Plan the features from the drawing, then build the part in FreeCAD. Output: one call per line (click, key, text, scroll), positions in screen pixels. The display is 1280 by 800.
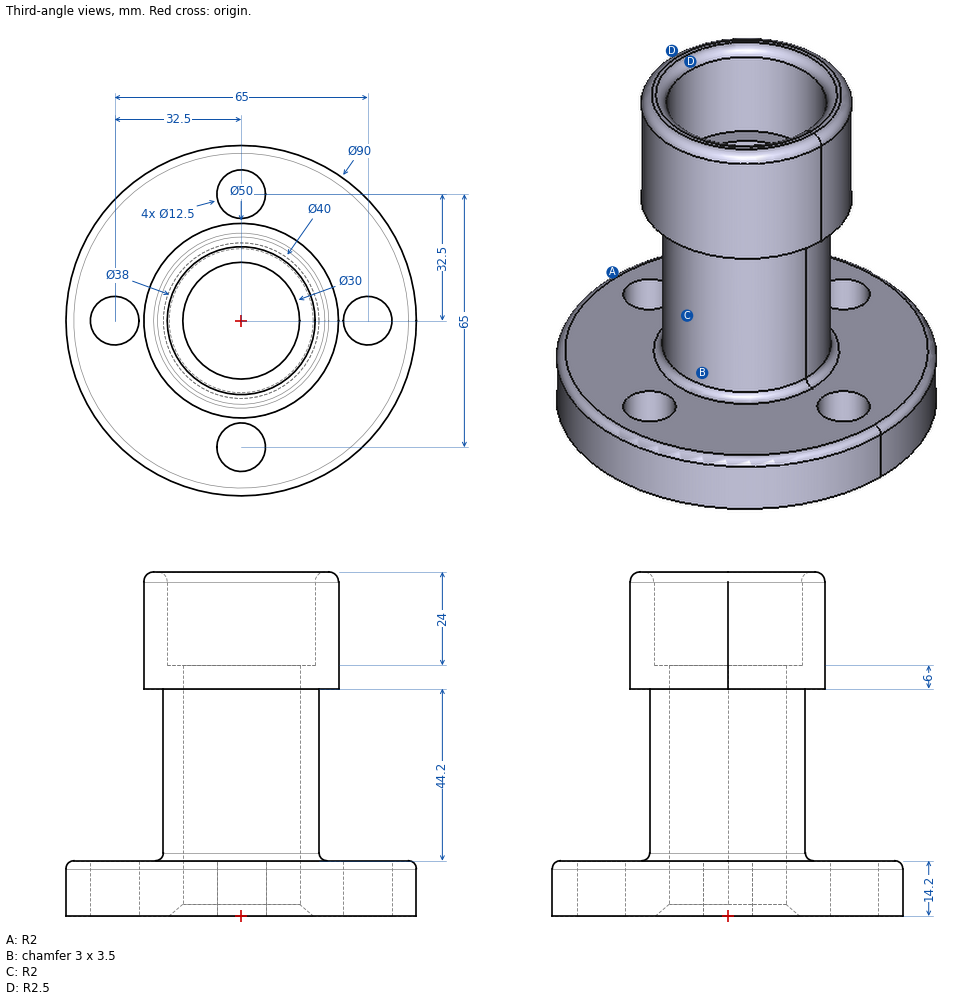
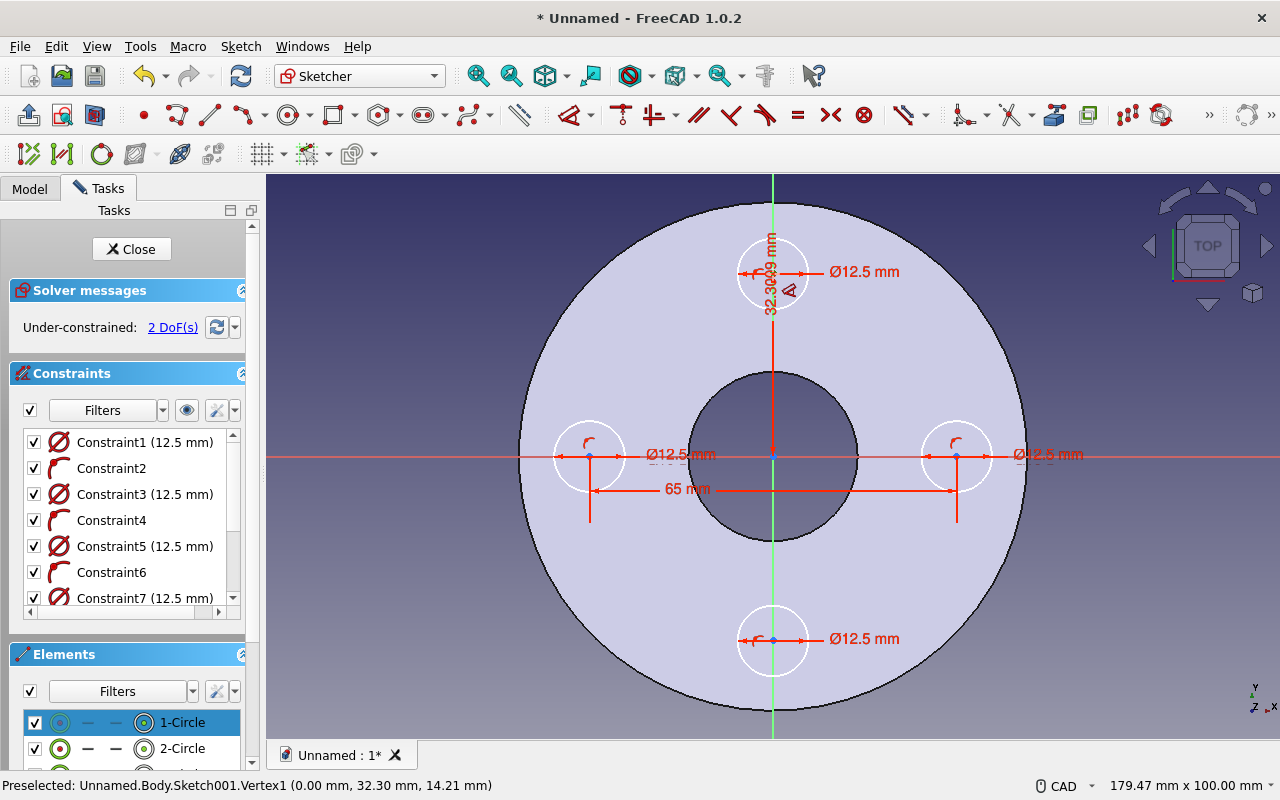
click(773, 641)
click(807, 373)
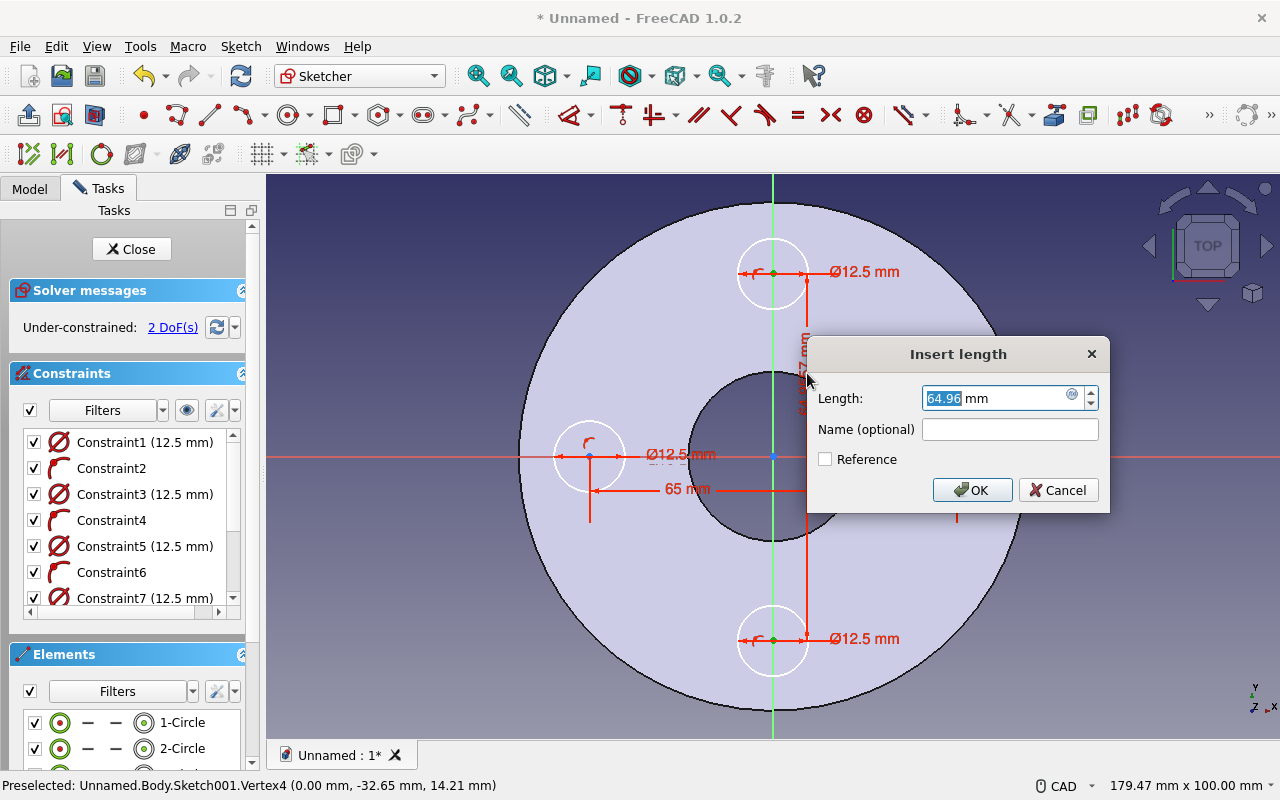
text(65)
key(Return)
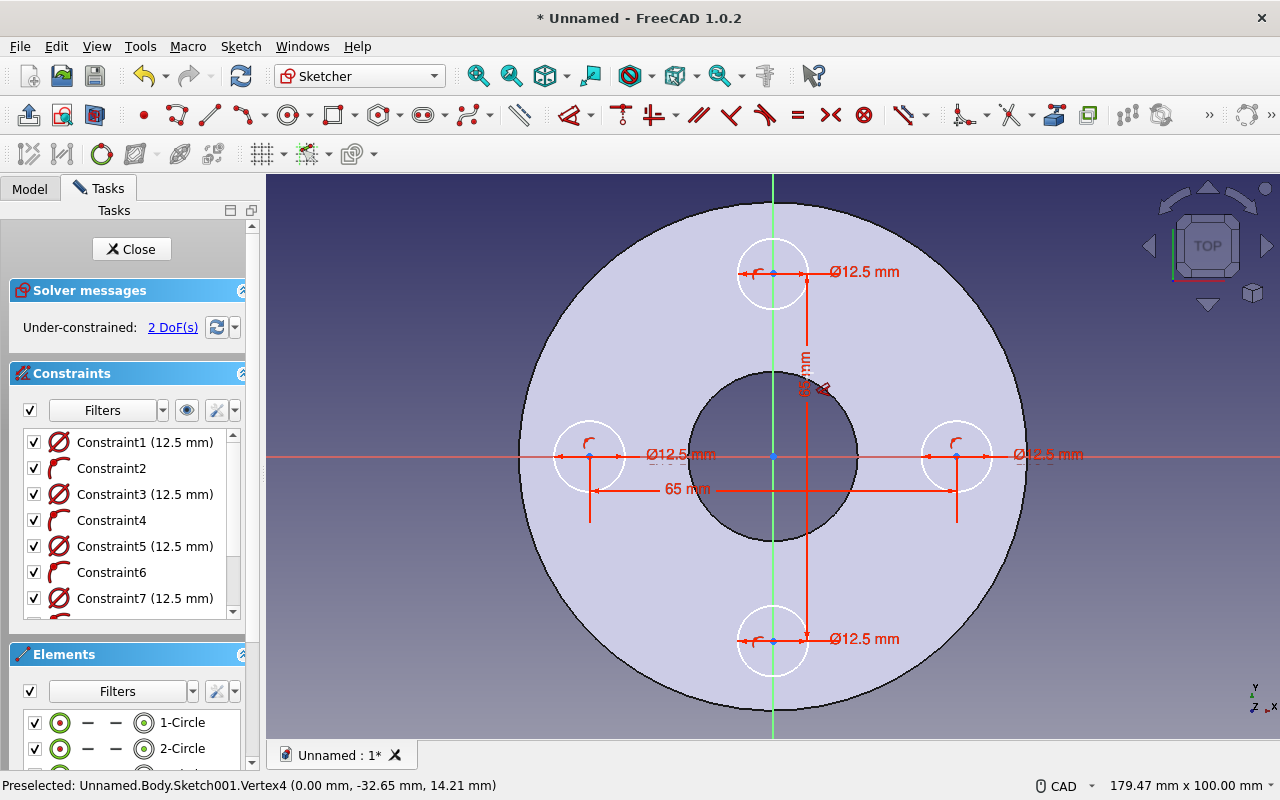
click(773, 274)
click(807, 323)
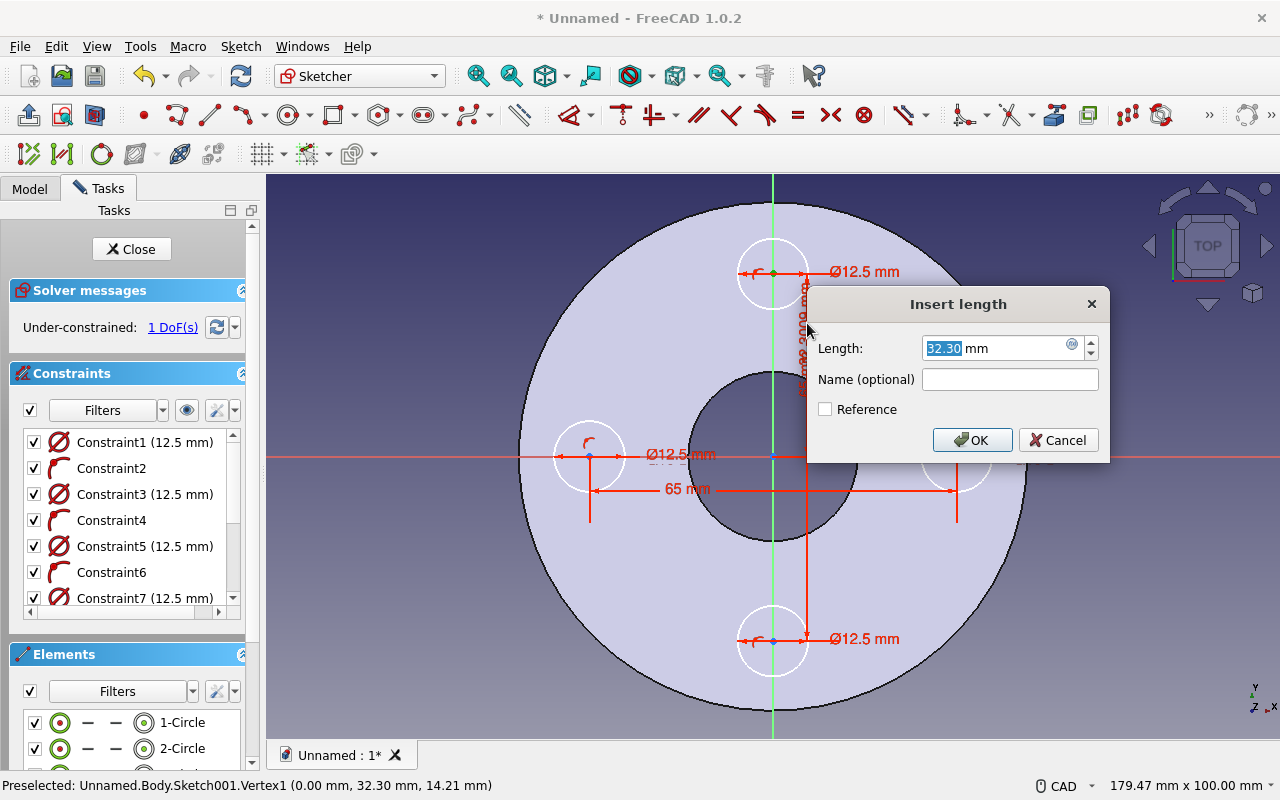
text(32.5)
key(Return)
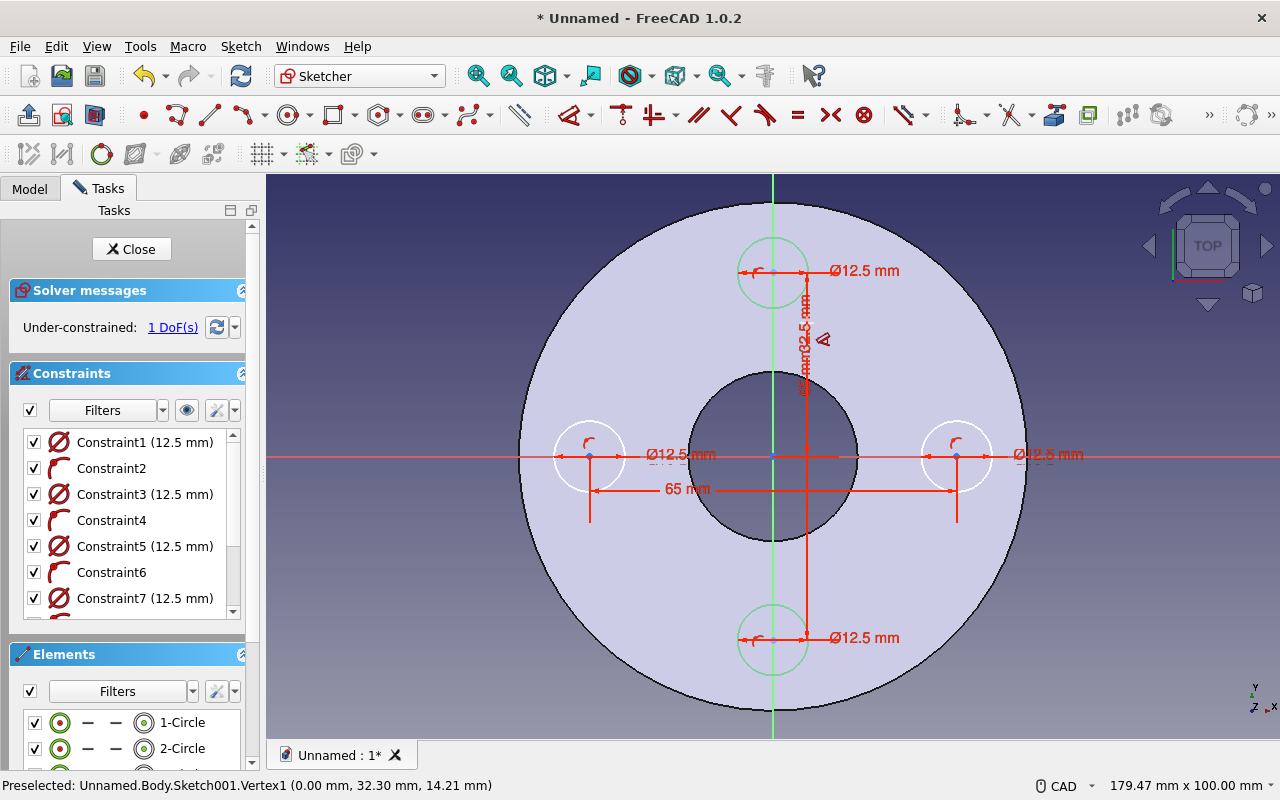
click(590, 456)
click(681, 422)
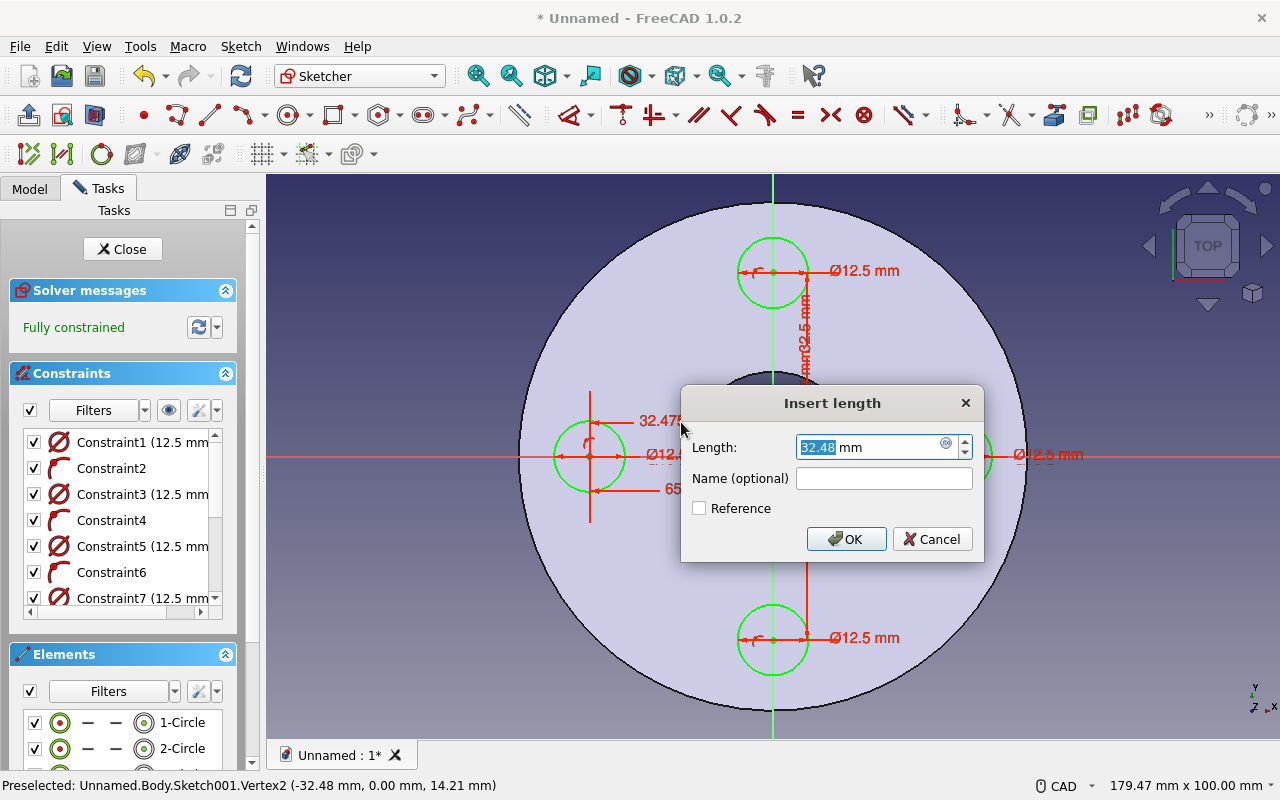
text(32.5)
key(Return)
key(Escape)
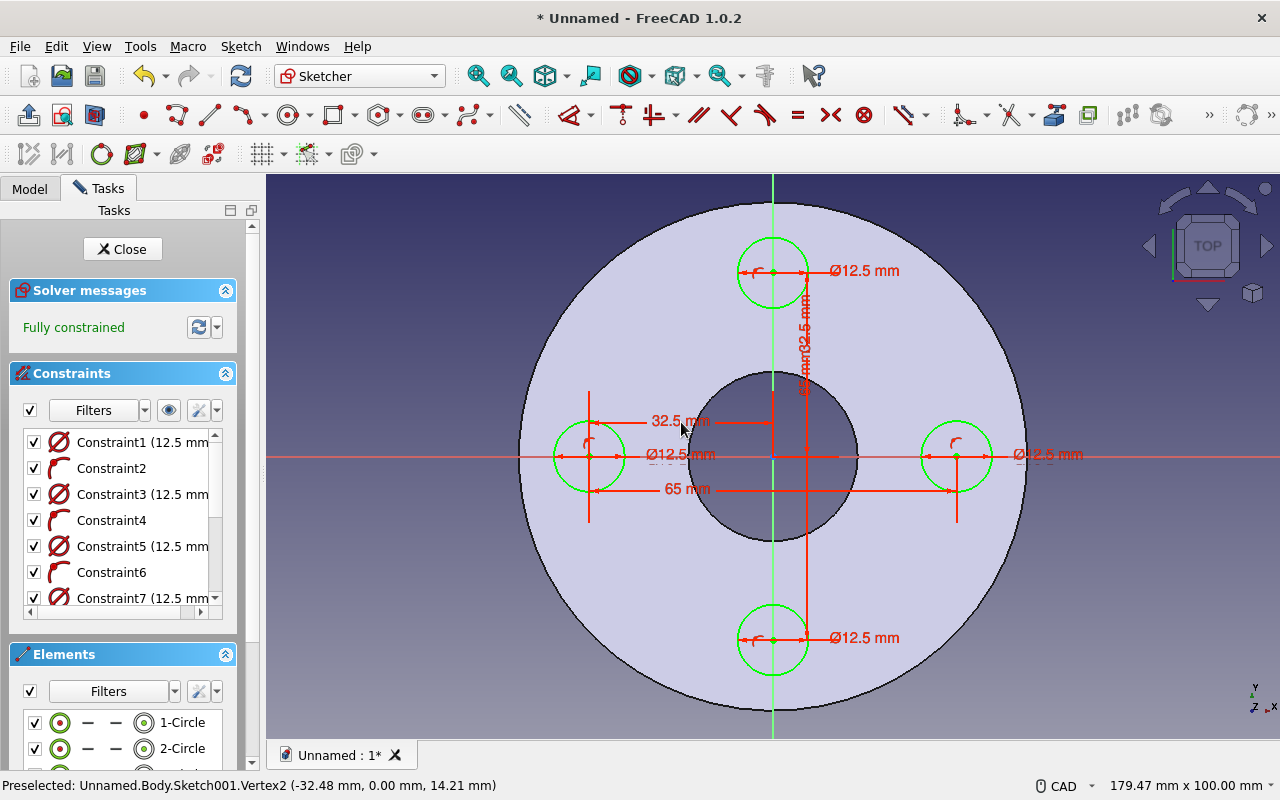
click(123, 249)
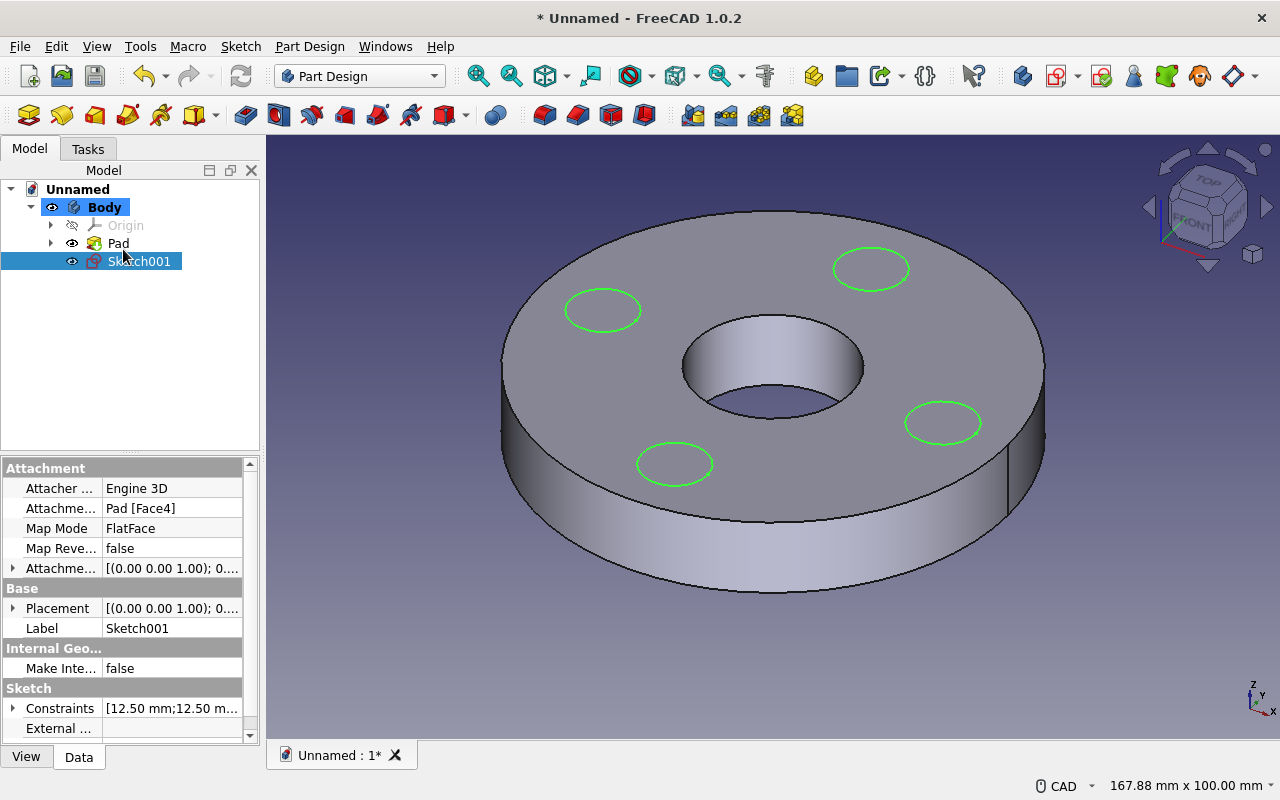
click(246, 116)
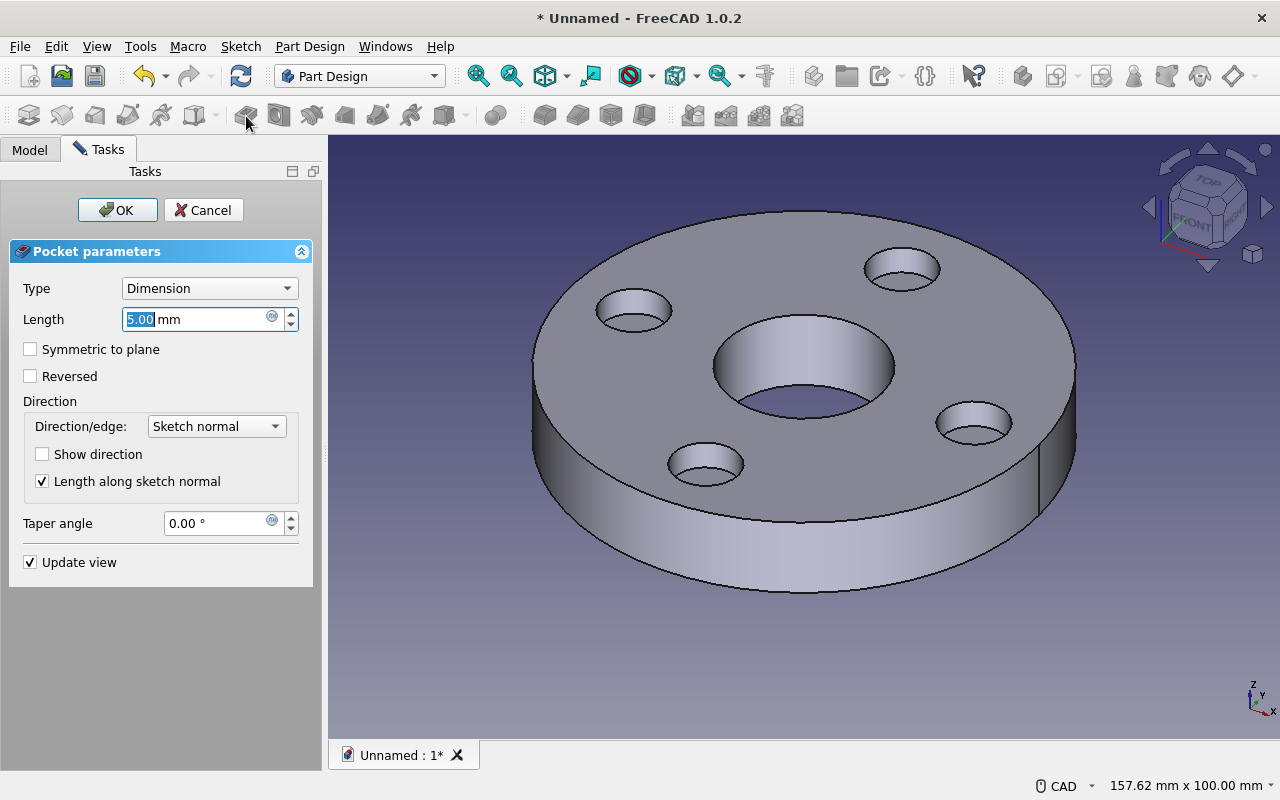
click(210, 288)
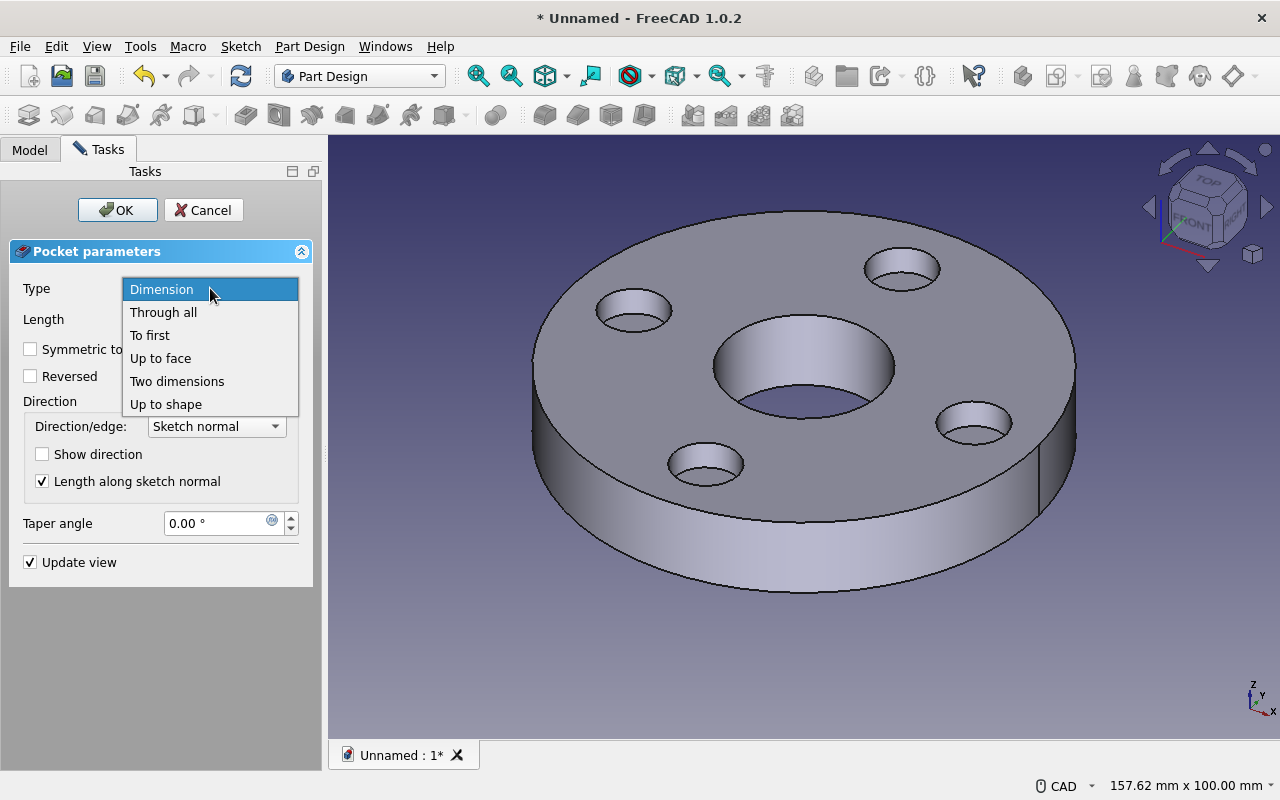
click(208, 312)